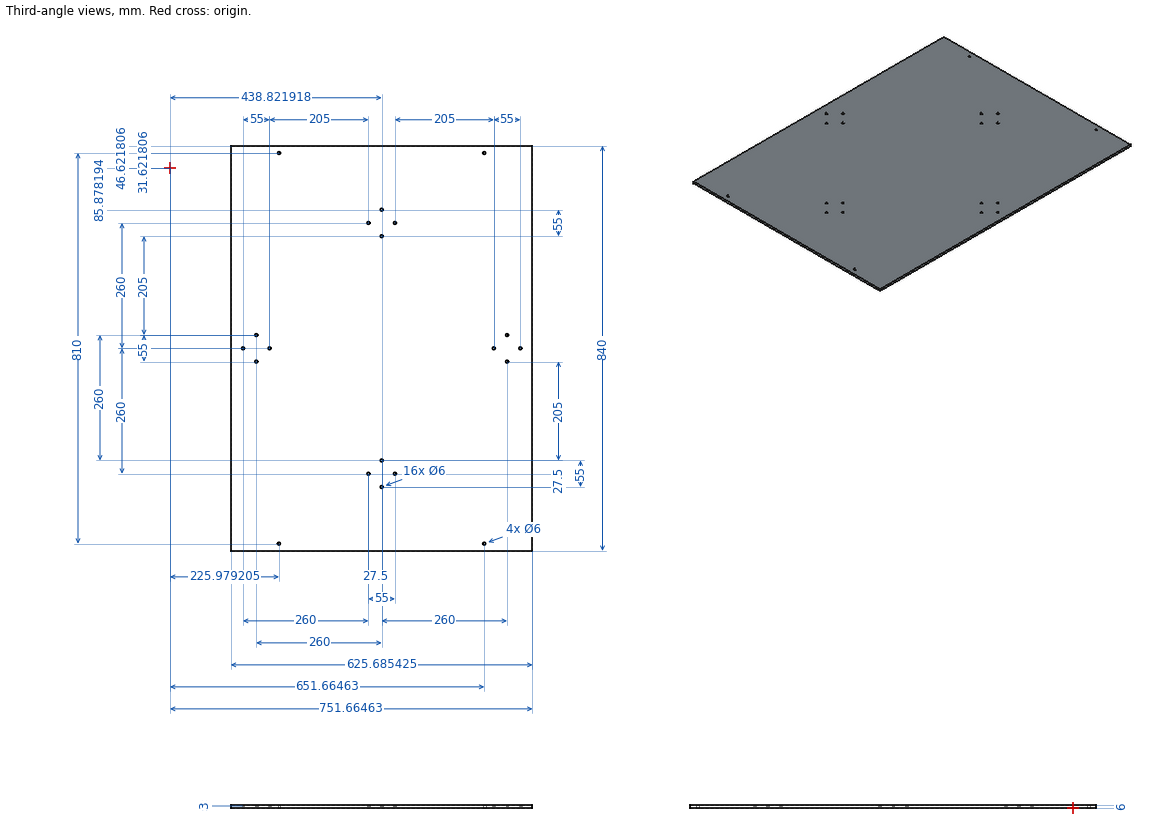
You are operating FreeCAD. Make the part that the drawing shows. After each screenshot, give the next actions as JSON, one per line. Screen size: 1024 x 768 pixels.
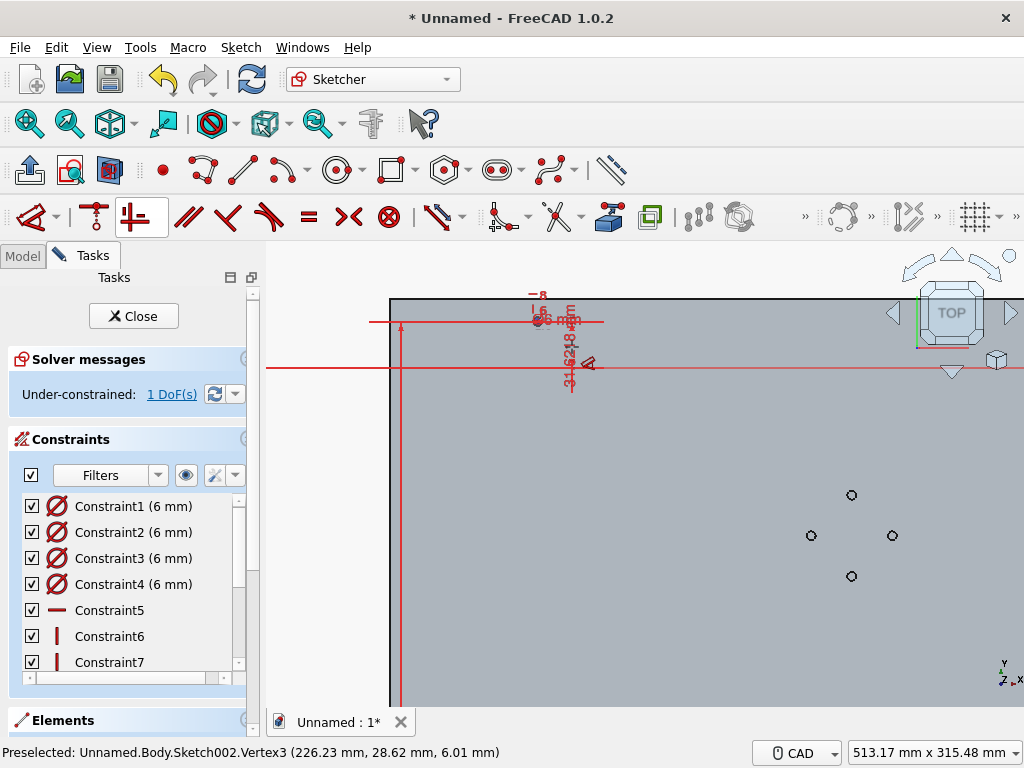
{"action": "scroll", "coordinate": [540, 328], "scroll_direction": "down", "scroll_amount": 7}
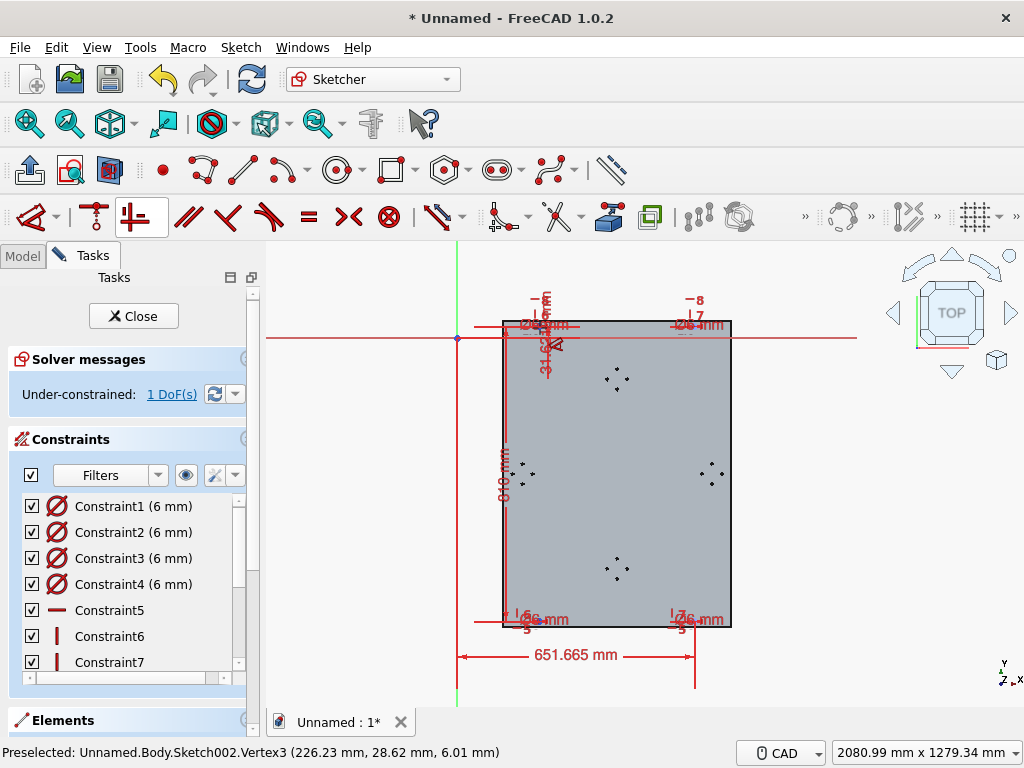
{"action": "left_click", "coordinate": [540, 622]}
{"action": "left_click", "coordinate": [499, 656]}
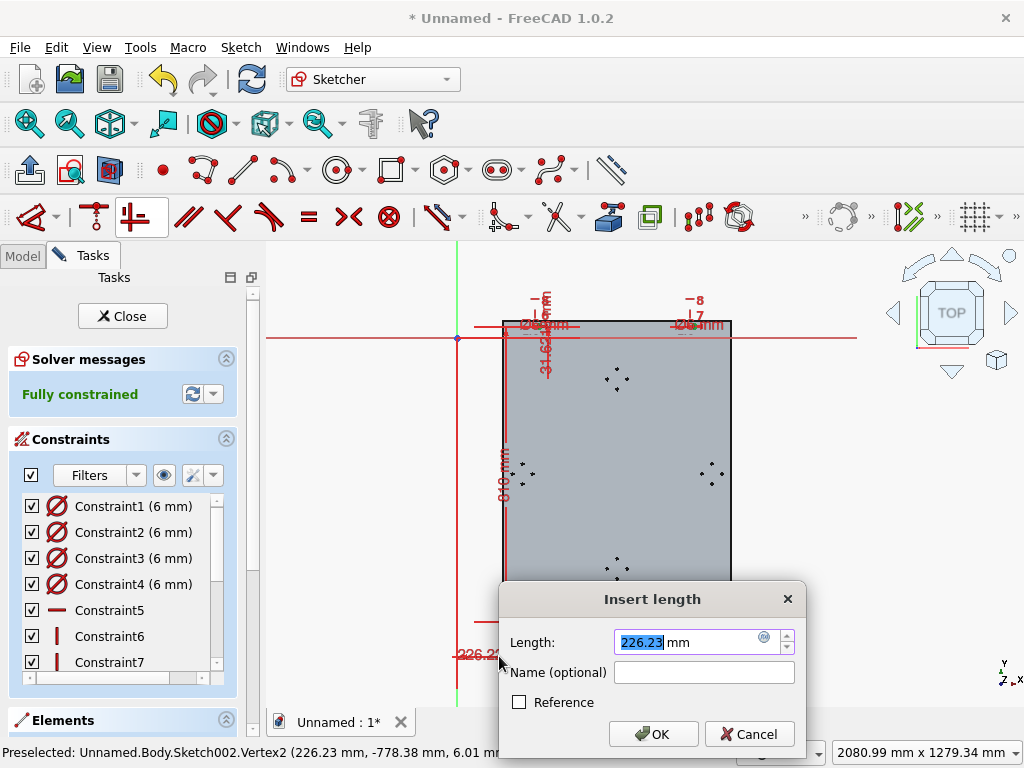
{"action": "type", "text": "225.979205"}
{"action": "key", "text": "Return"}
{"action": "key", "text": "Escape"}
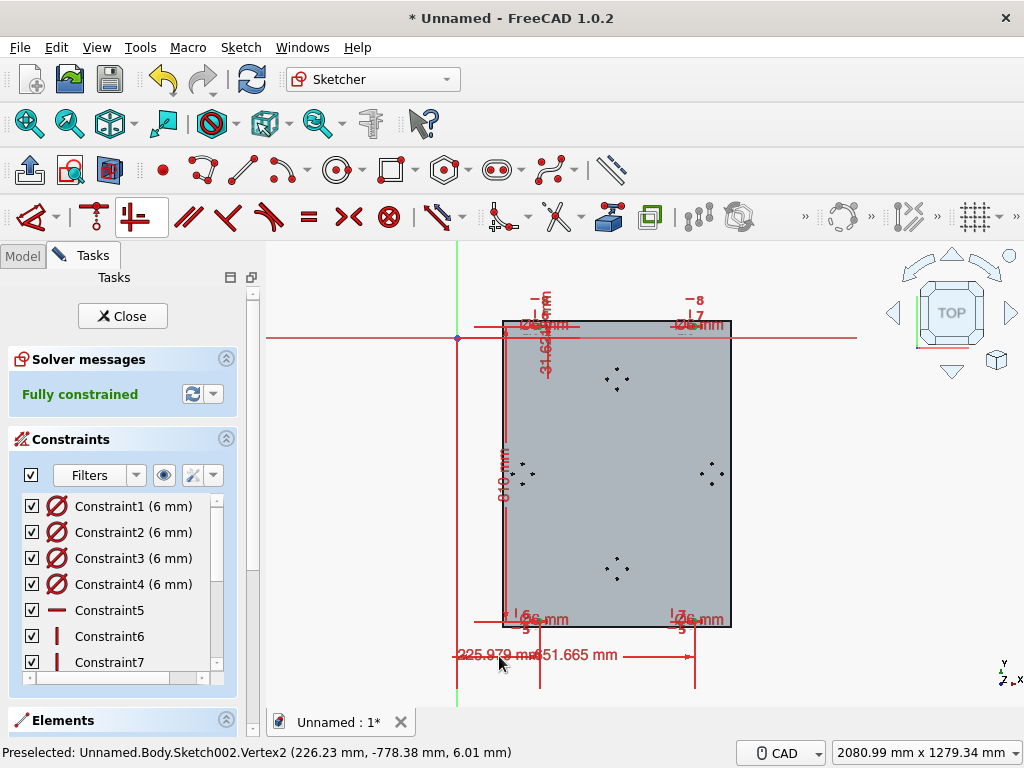
{"action": "left_click", "coordinate": [123, 316]}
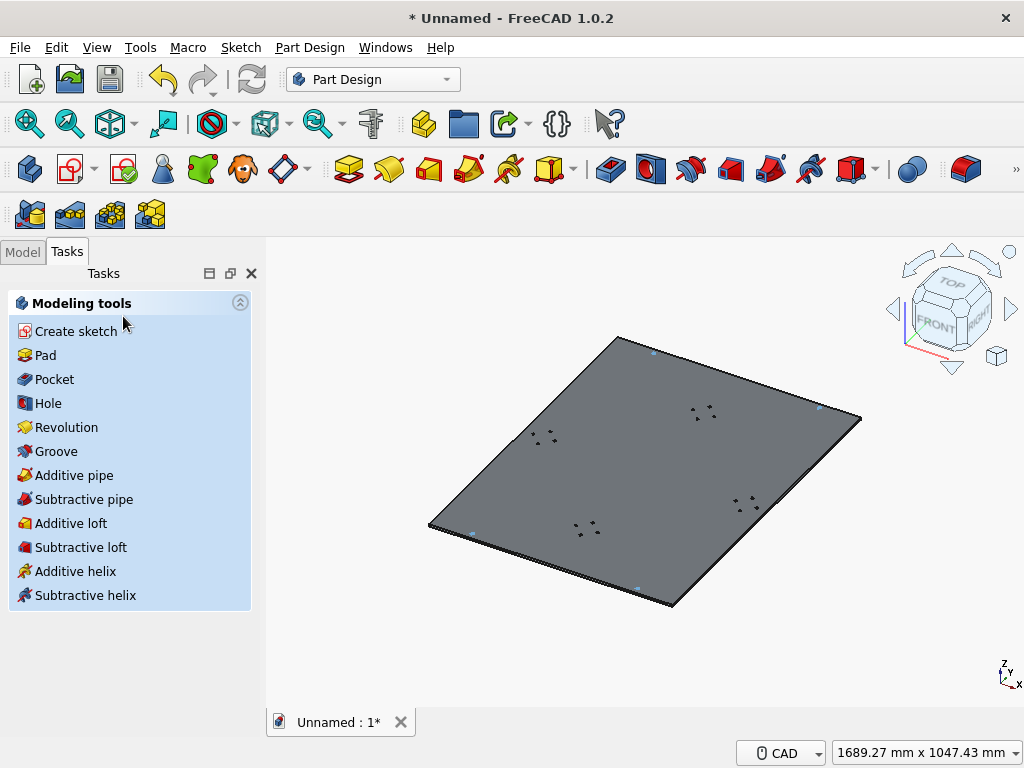
{"action": "left_click", "coordinate": [612, 170]}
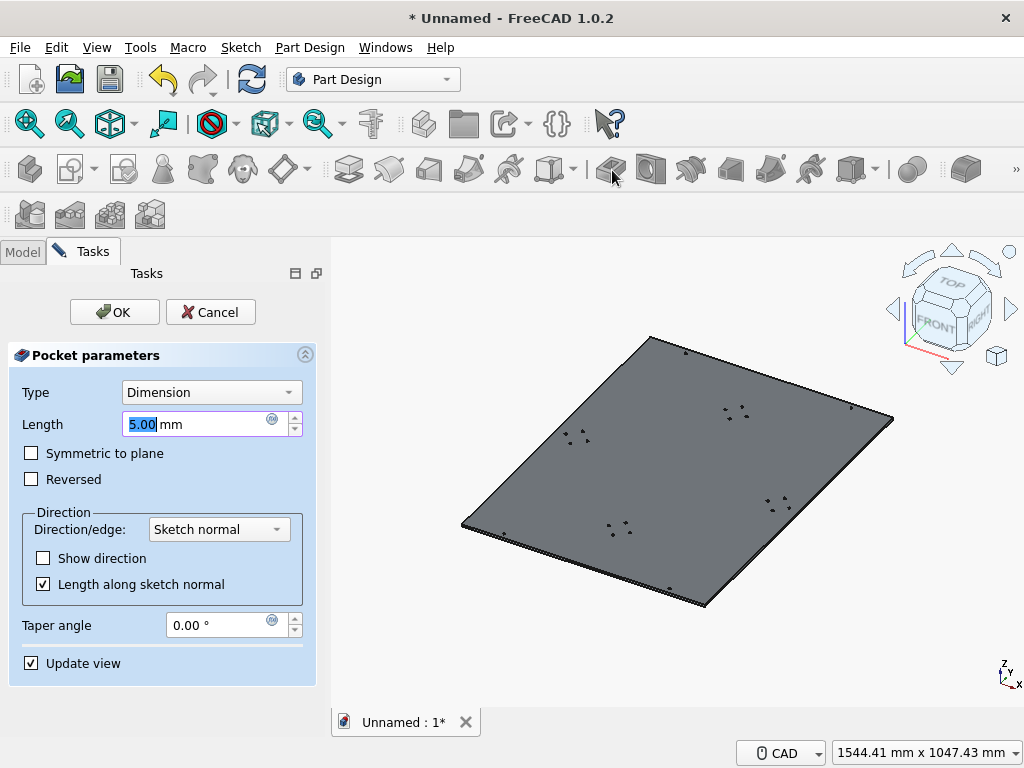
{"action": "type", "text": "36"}
{"action": "key", "text": "Tab"}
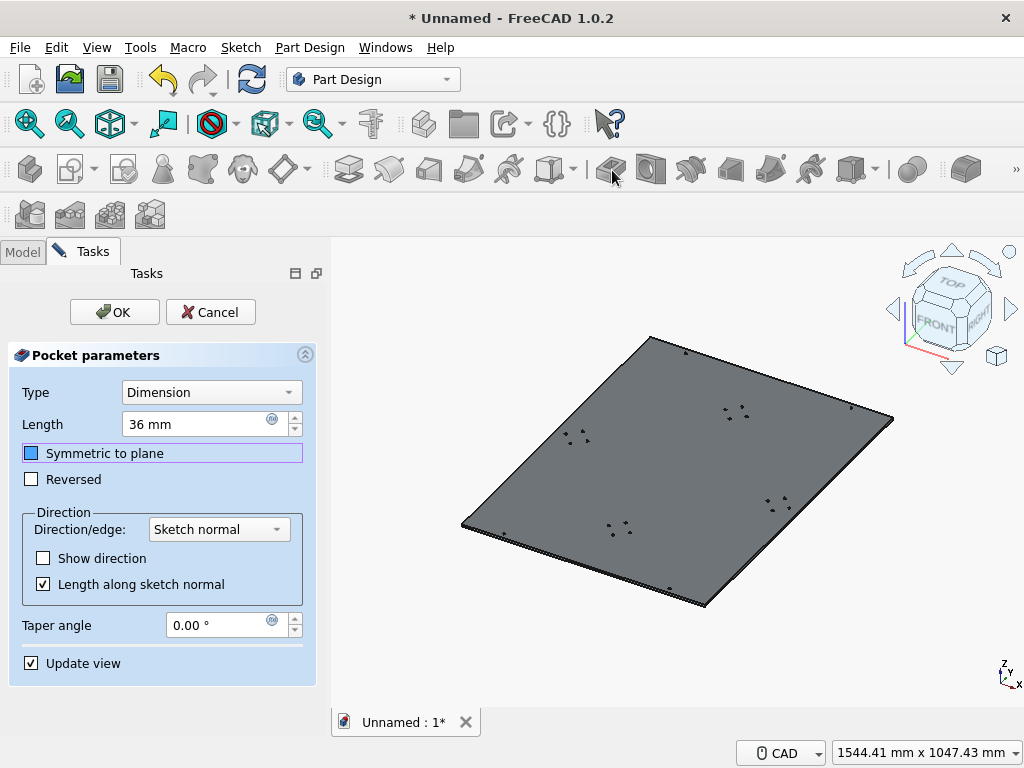
{"action": "left_click", "coordinate": [115, 312]}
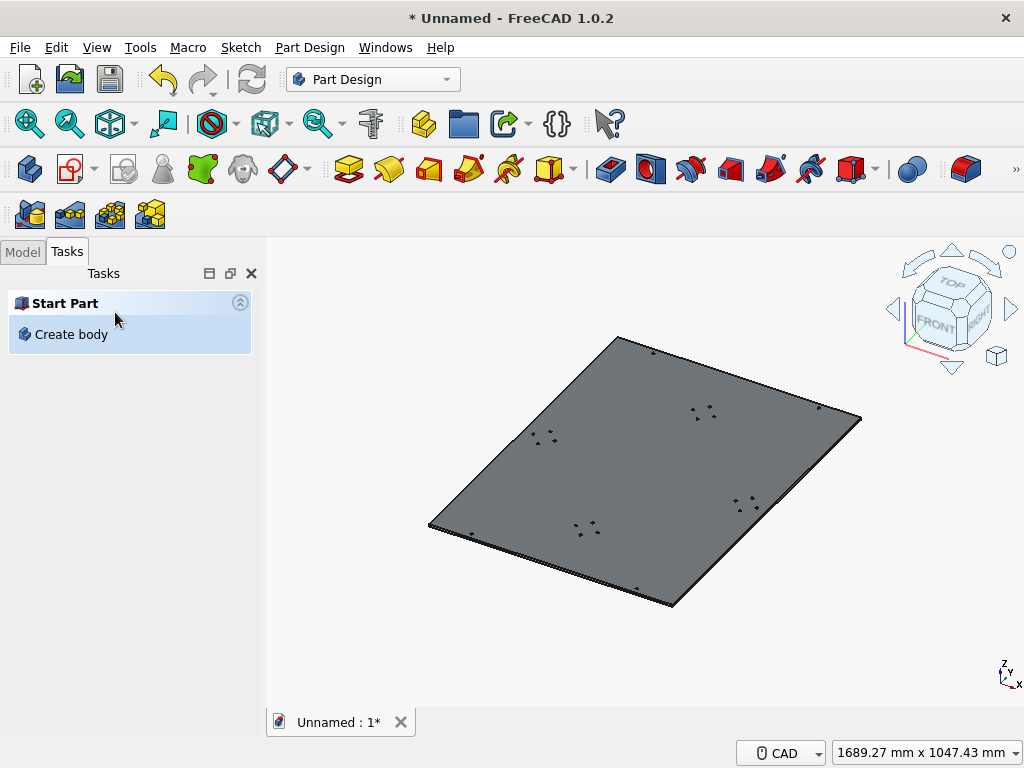
{"action": "key", "text": "0"}